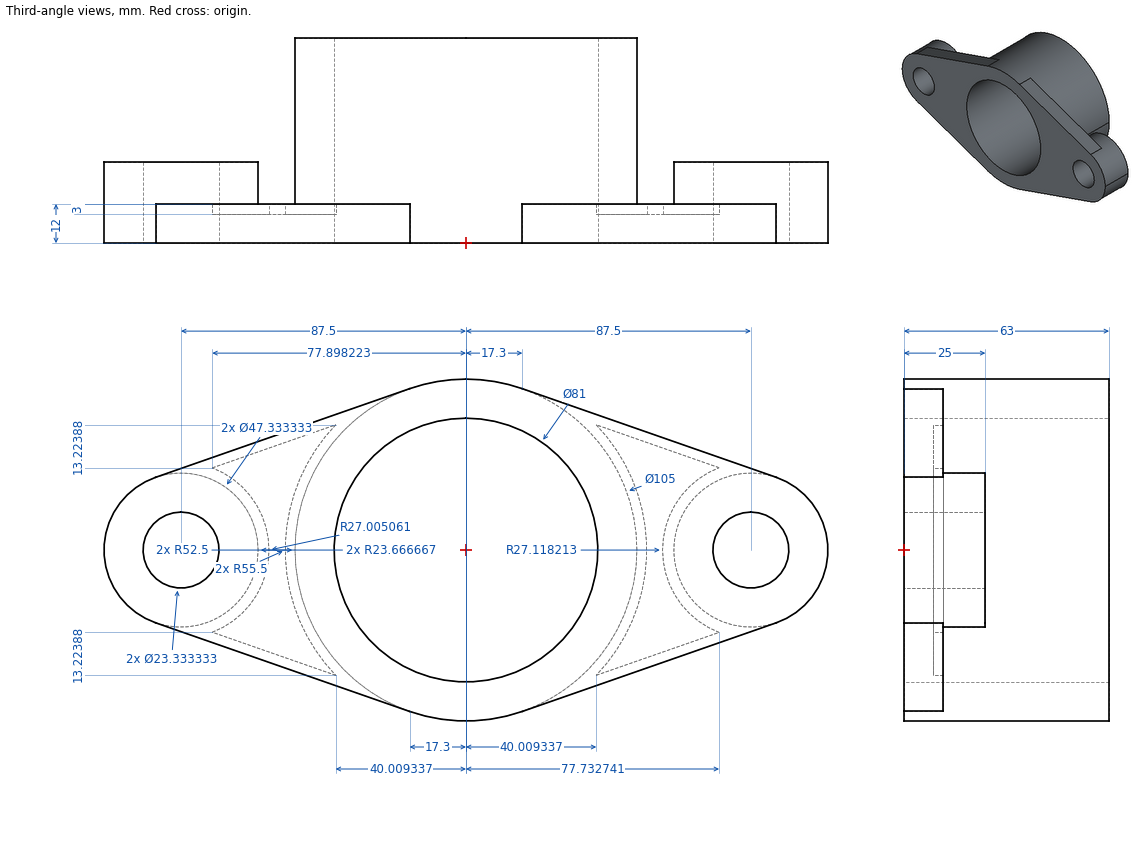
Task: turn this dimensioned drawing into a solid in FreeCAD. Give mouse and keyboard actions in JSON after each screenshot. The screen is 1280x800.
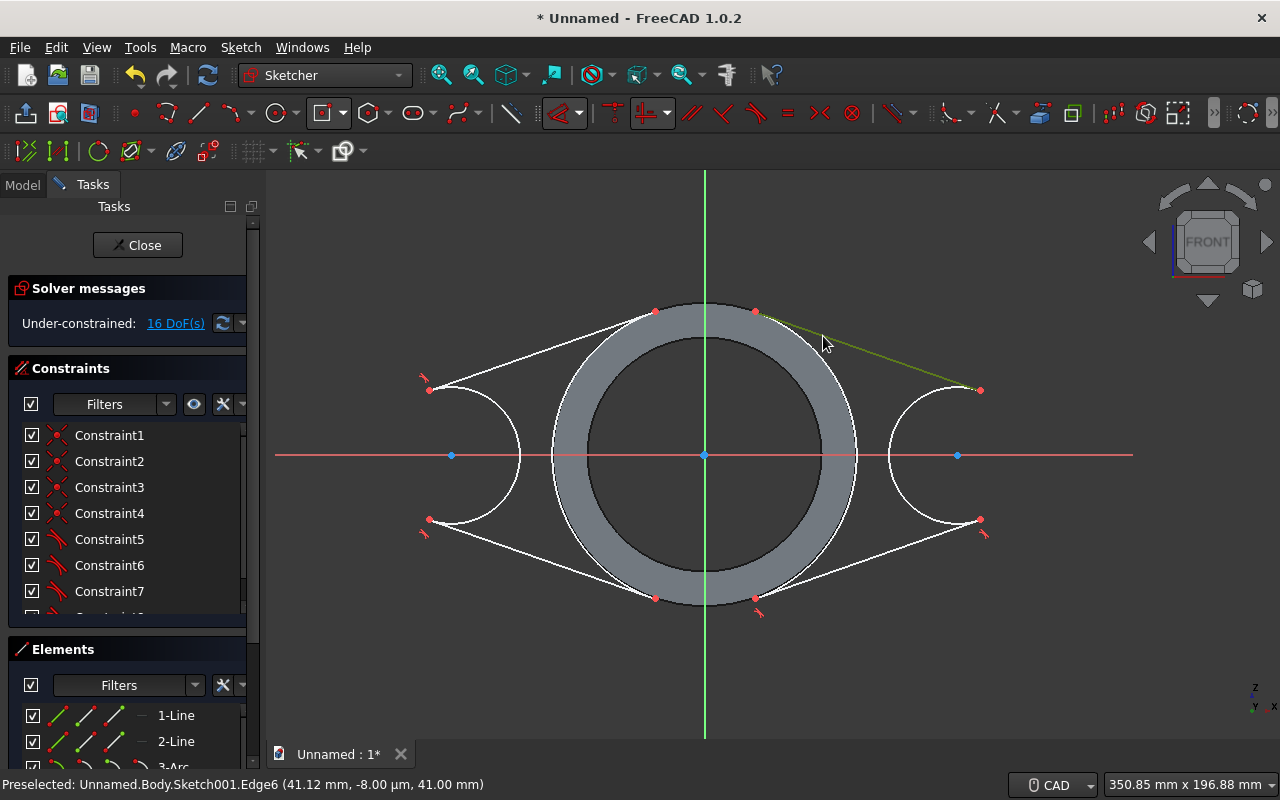
{"action": "left_click", "coordinate": [908, 408]}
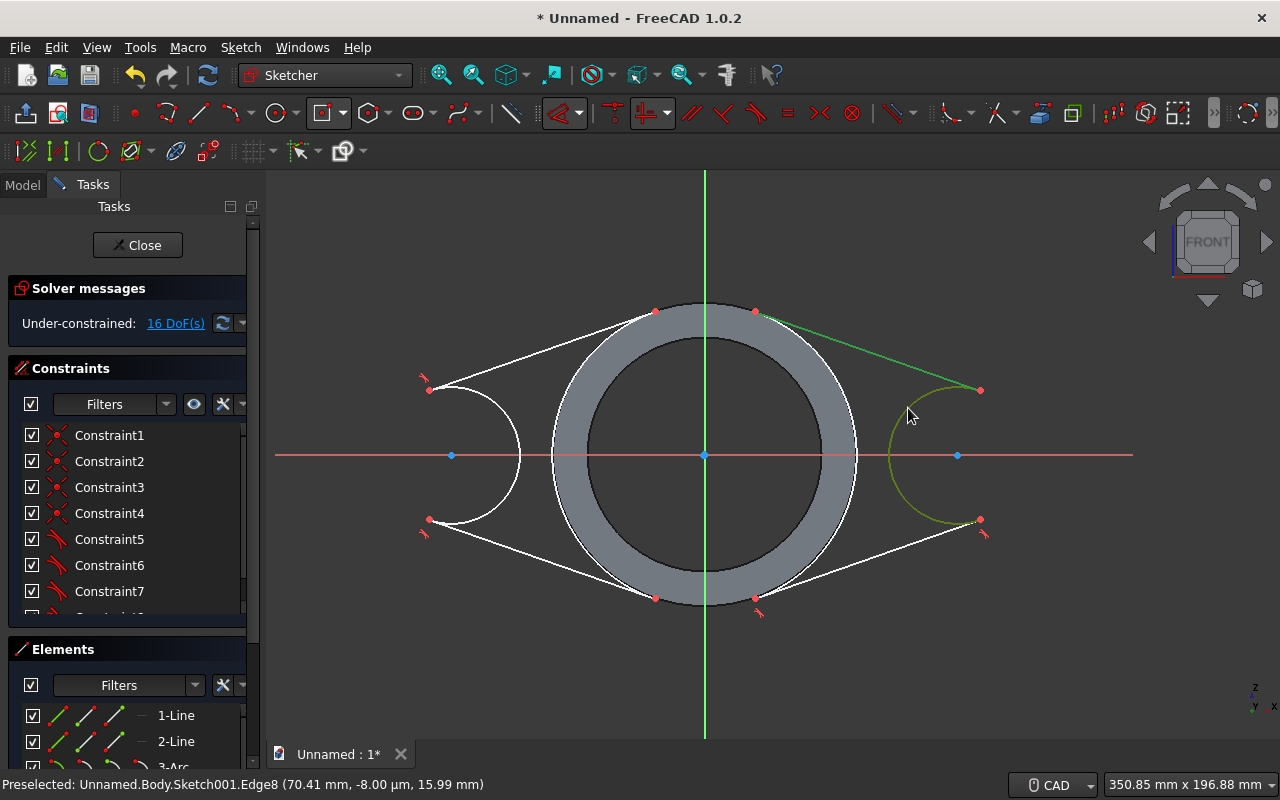
{"action": "key", "text": "t"}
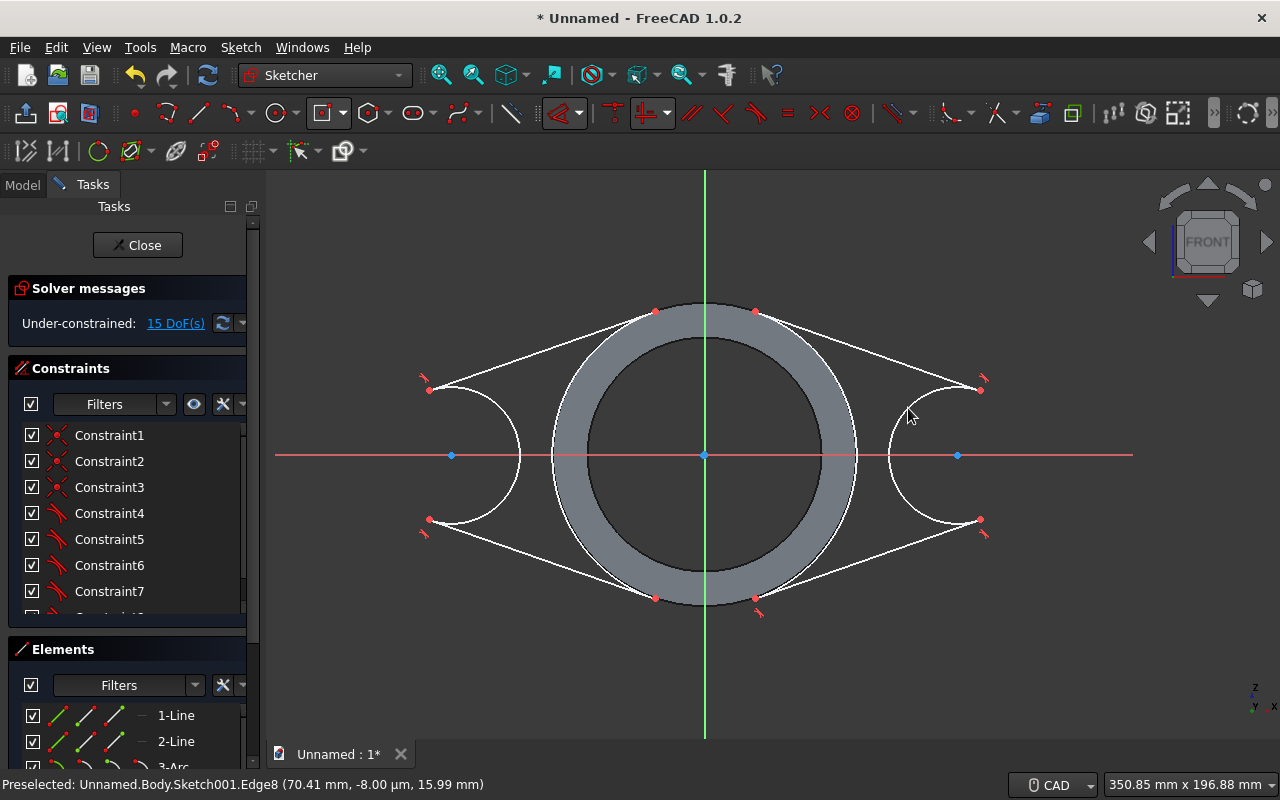
{"action": "left_click", "coordinate": [571, 383]}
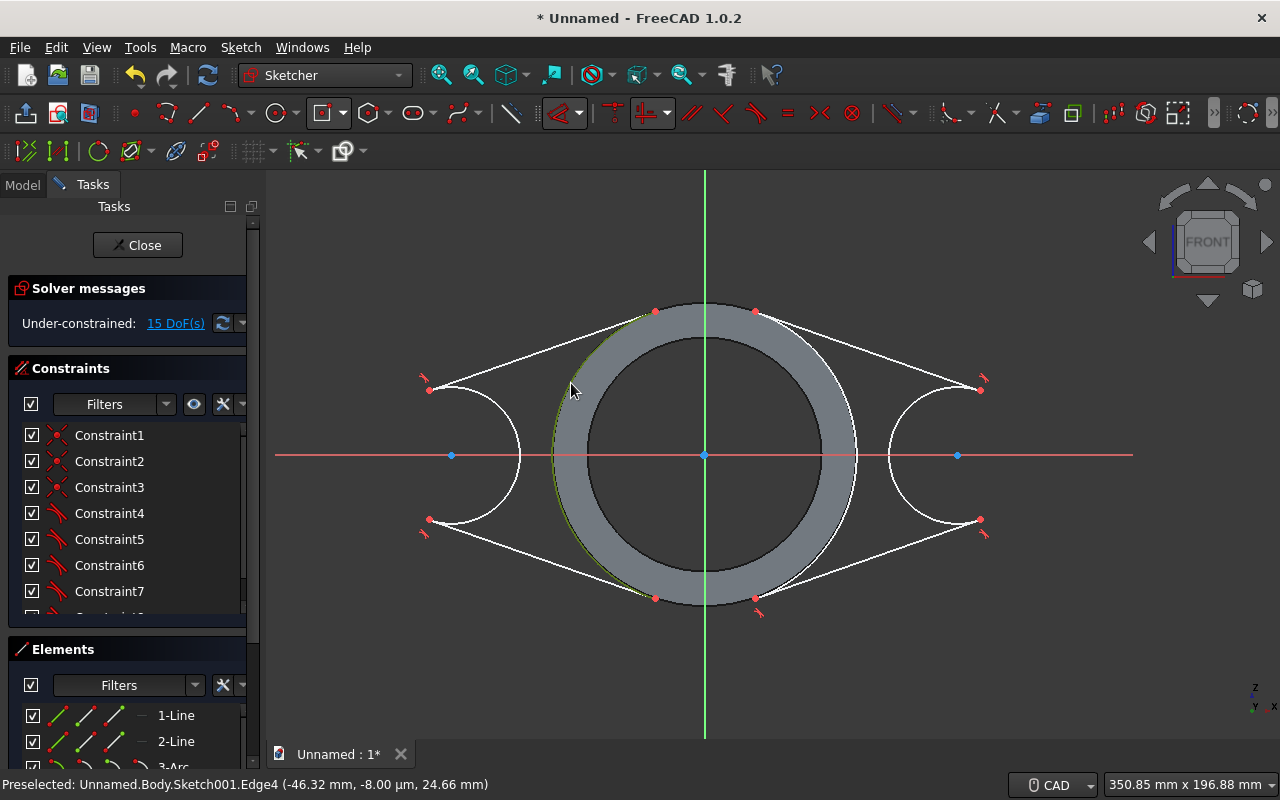
{"action": "left_click", "coordinate": [839, 528]}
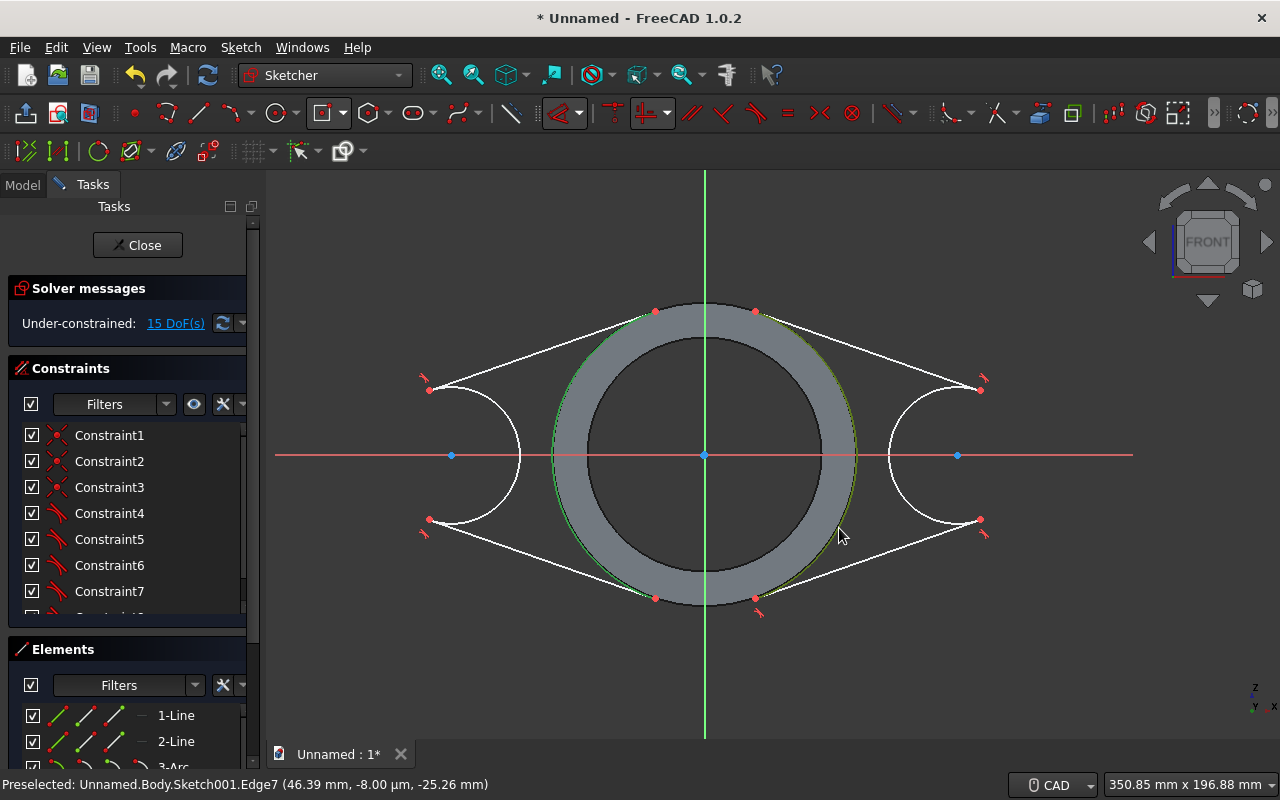
{"action": "key", "text": "c"}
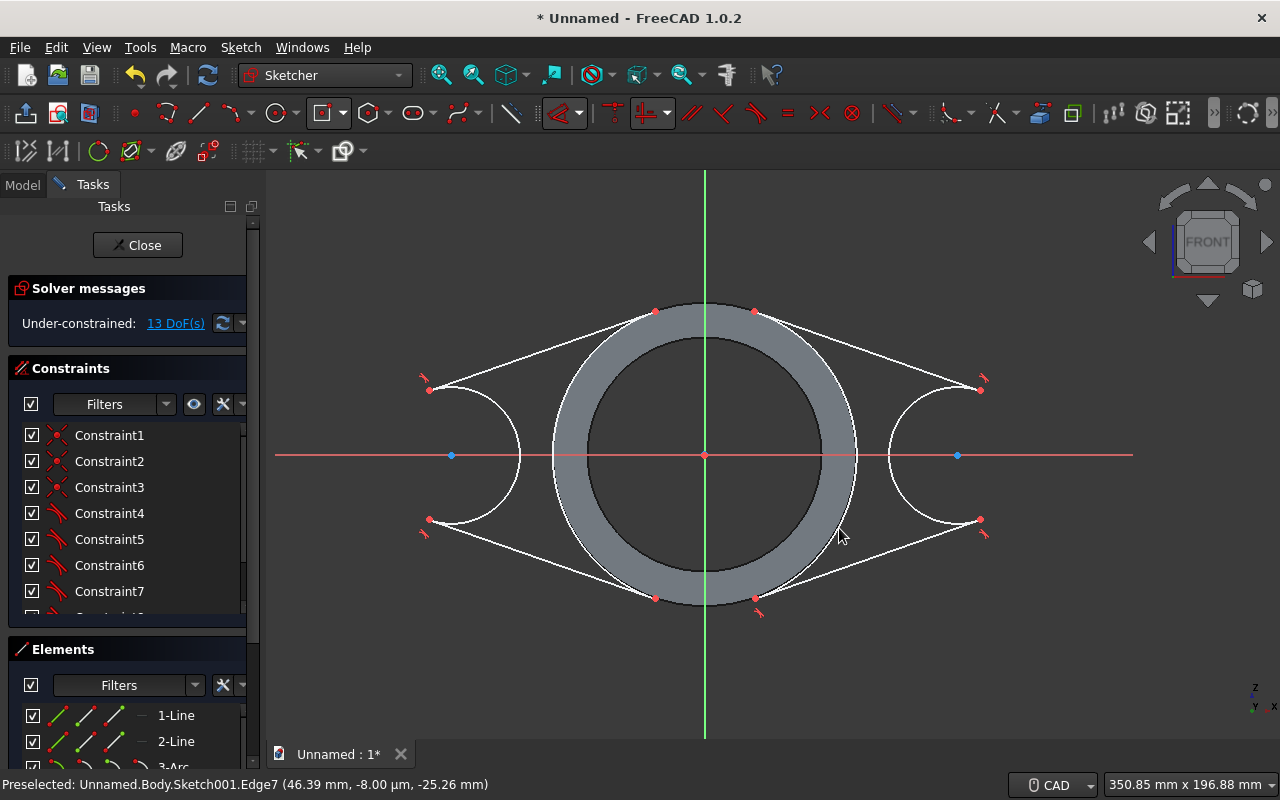
{"action": "left_click_drag", "start_coordinate": [695, 445], "coordinate": [715, 466]}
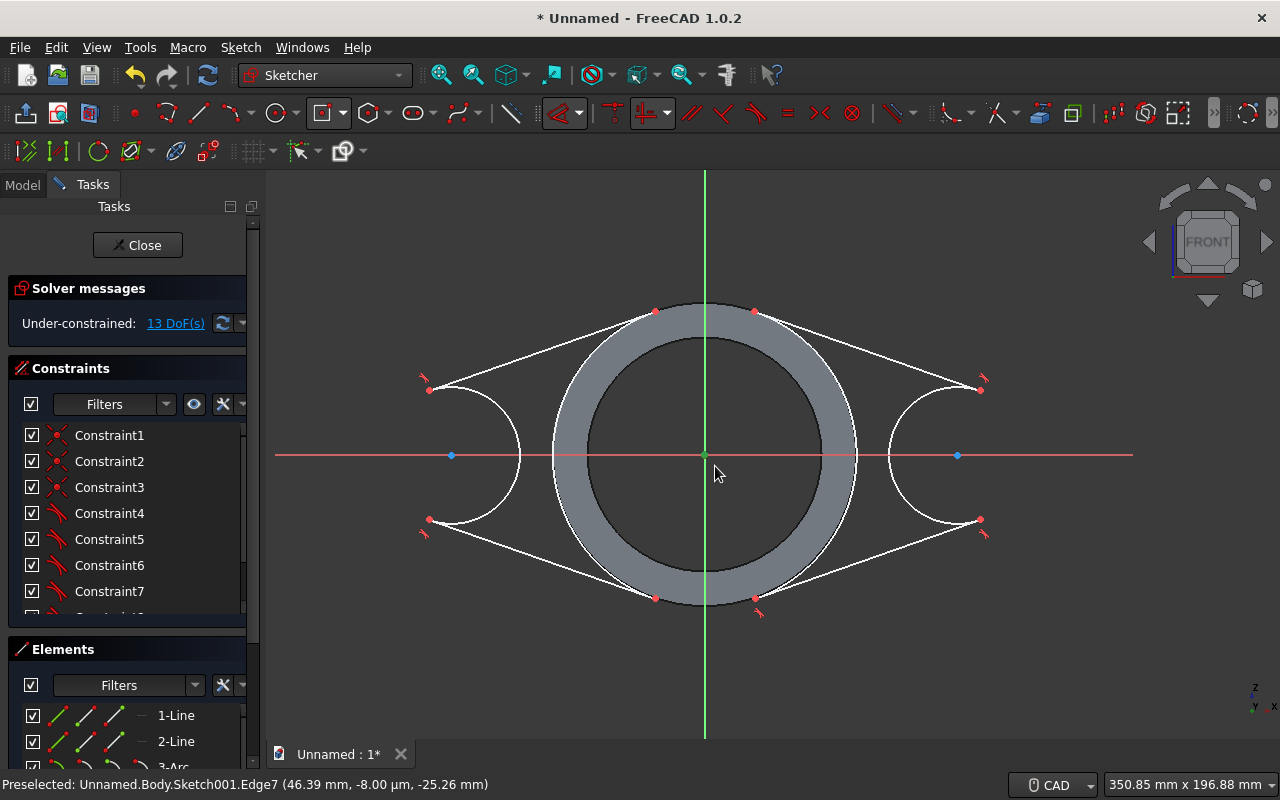
{"action": "left_click", "coordinate": [614, 114]}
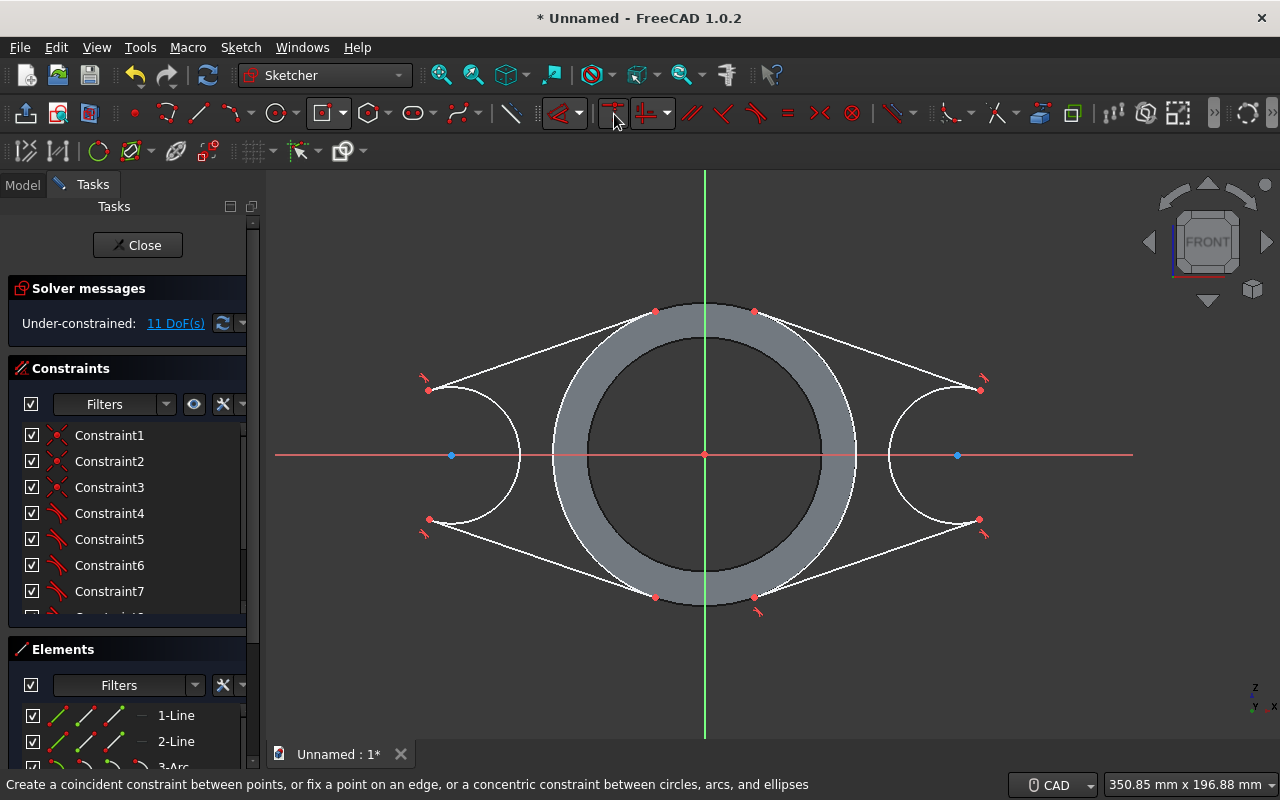
{"action": "left_click", "coordinate": [571, 383]}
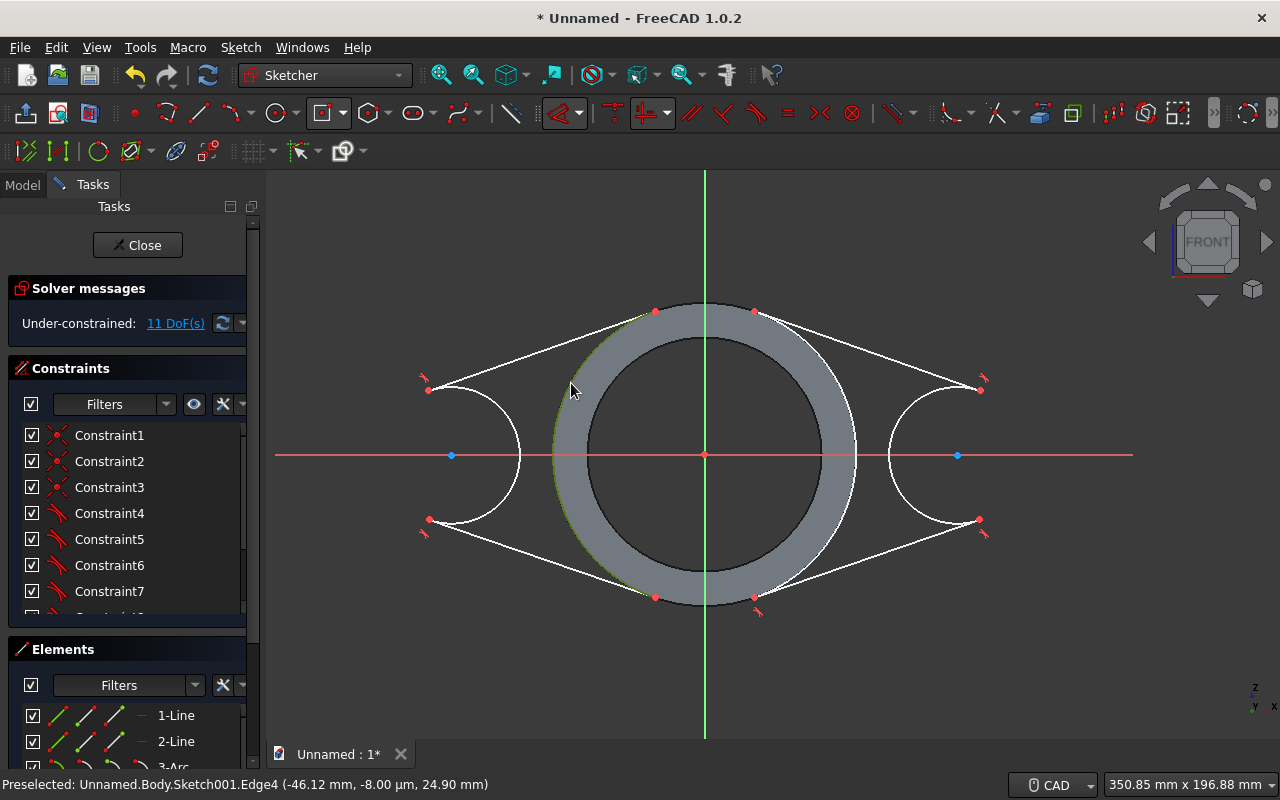
{"action": "left_click", "coordinate": [838, 527]}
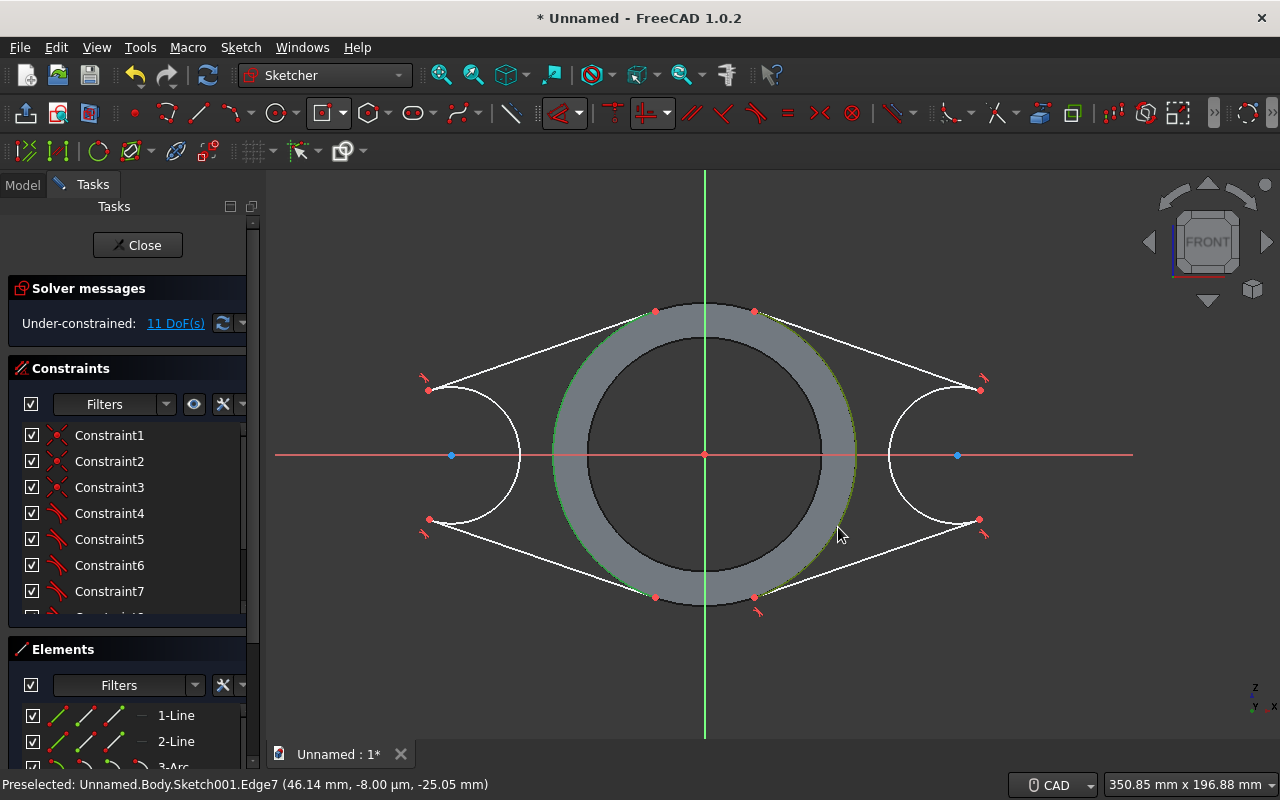
{"action": "key", "text": "e"}